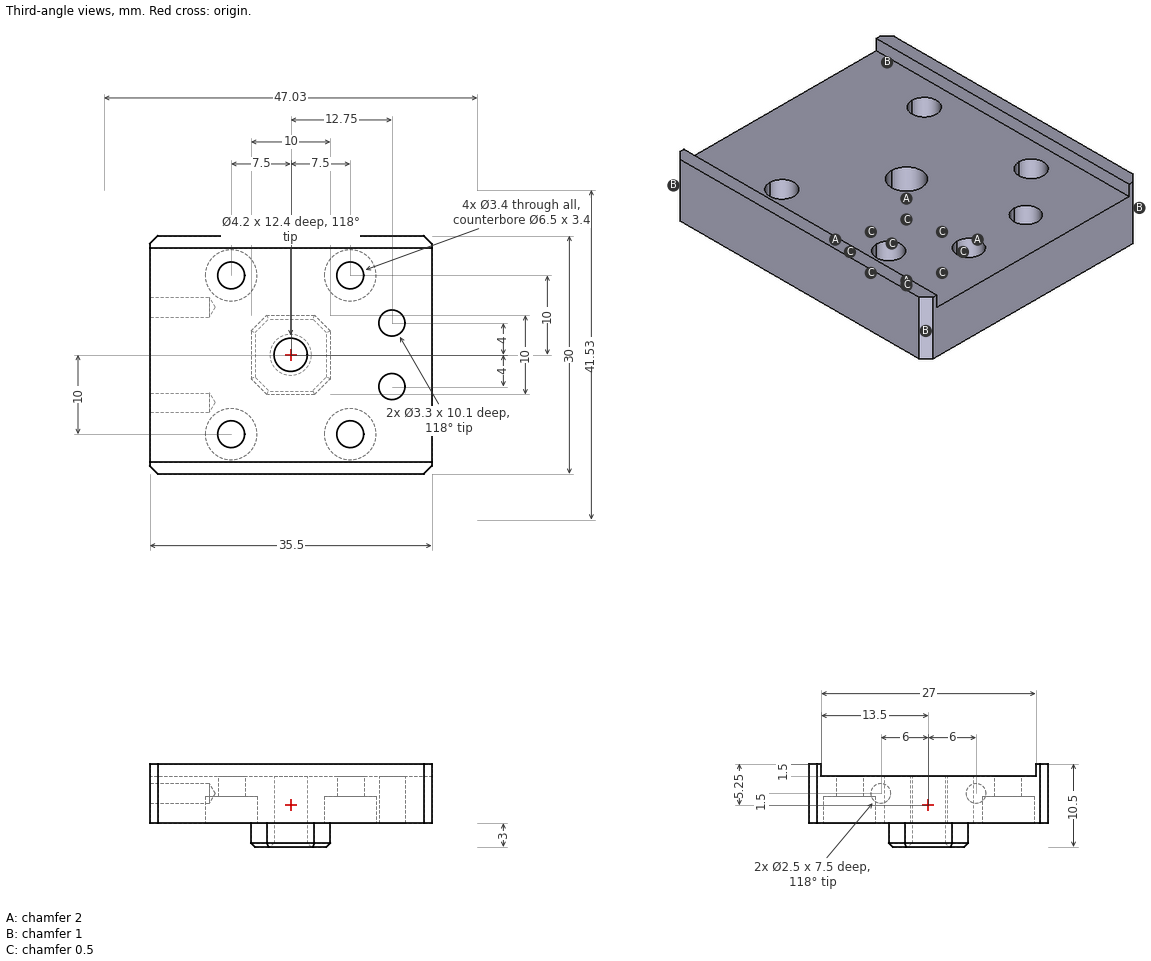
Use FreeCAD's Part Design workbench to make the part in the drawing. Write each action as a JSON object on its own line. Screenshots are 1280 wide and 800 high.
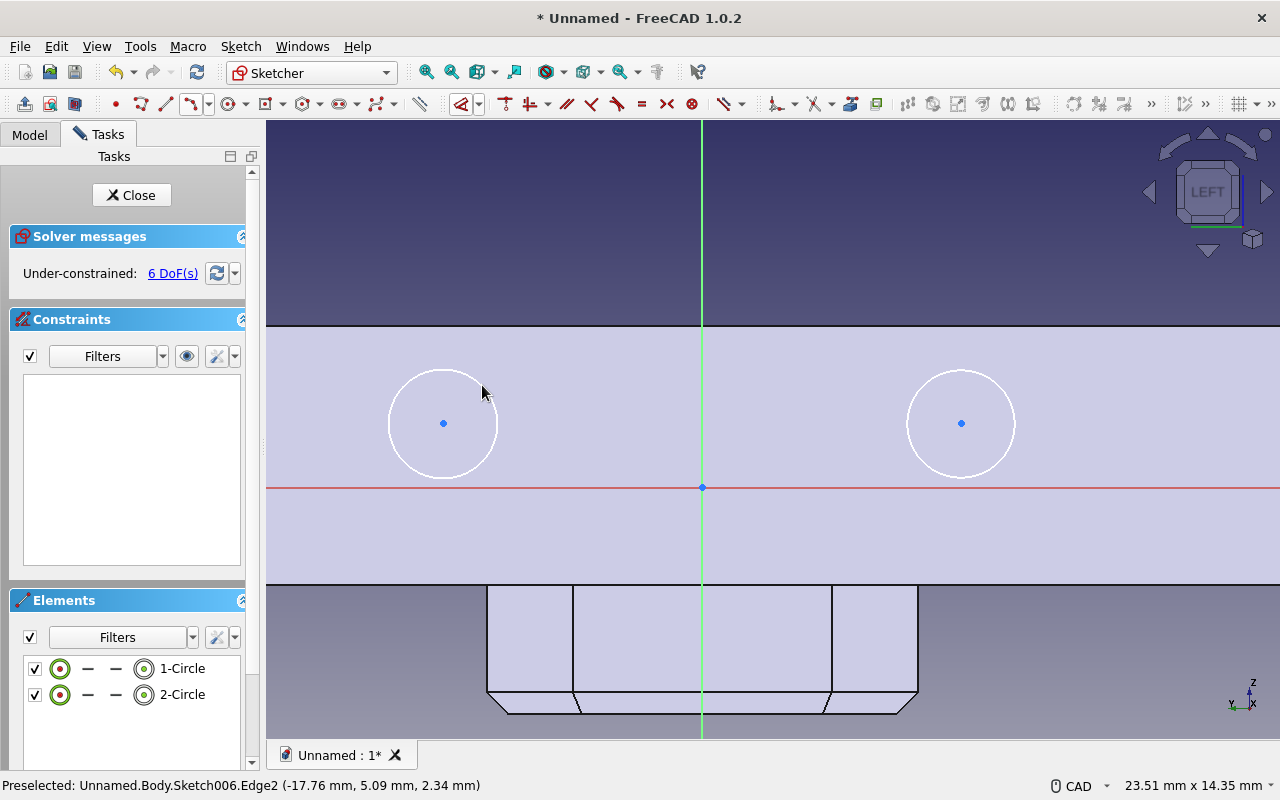
{"action": "left_click", "coordinate": [999, 386]}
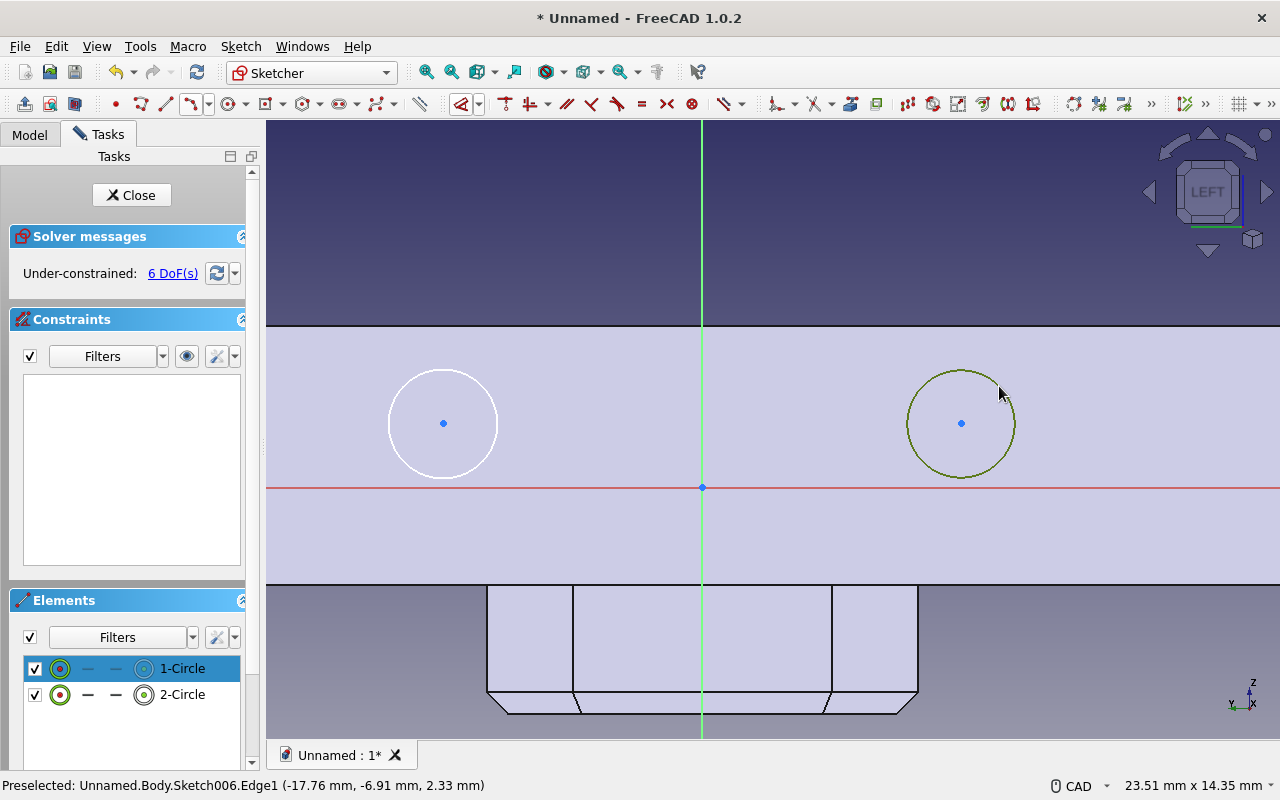
{"action": "left_click", "coordinate": [481, 385]}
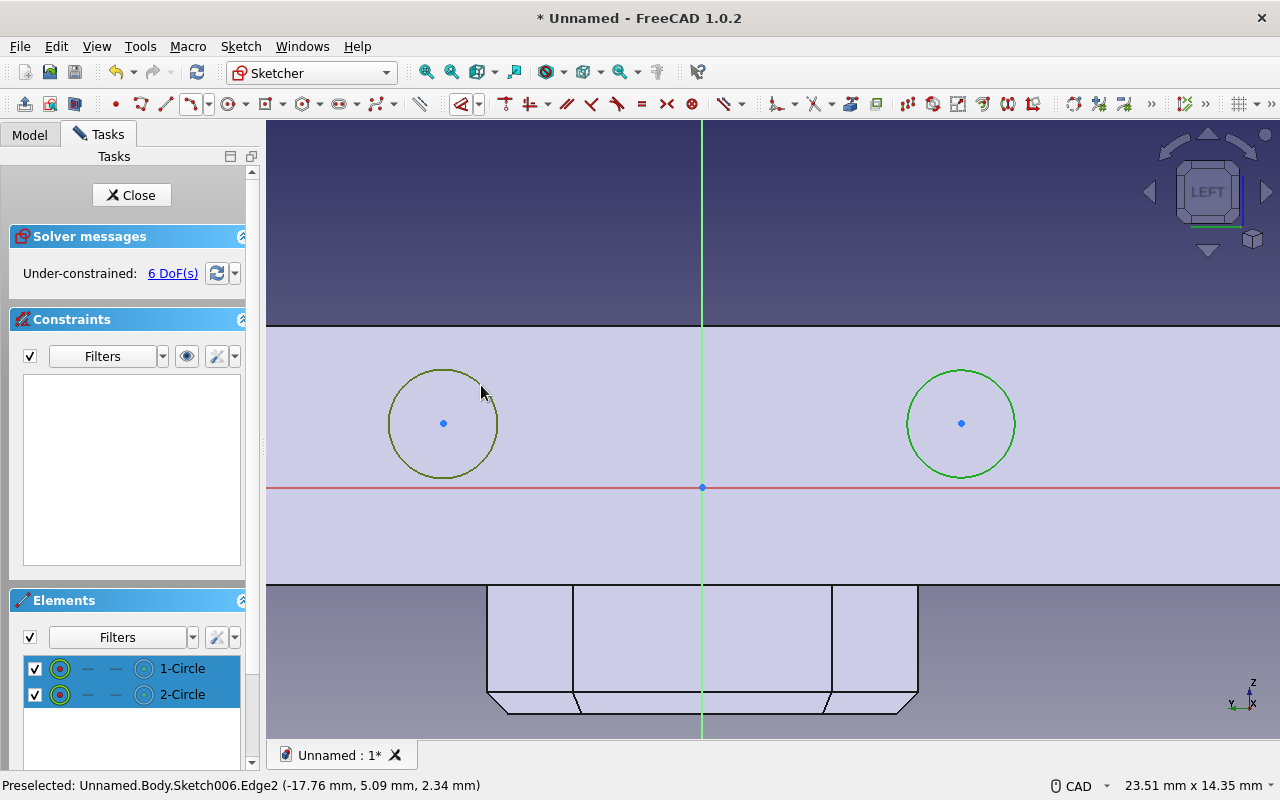
{"action": "key", "text": "e"}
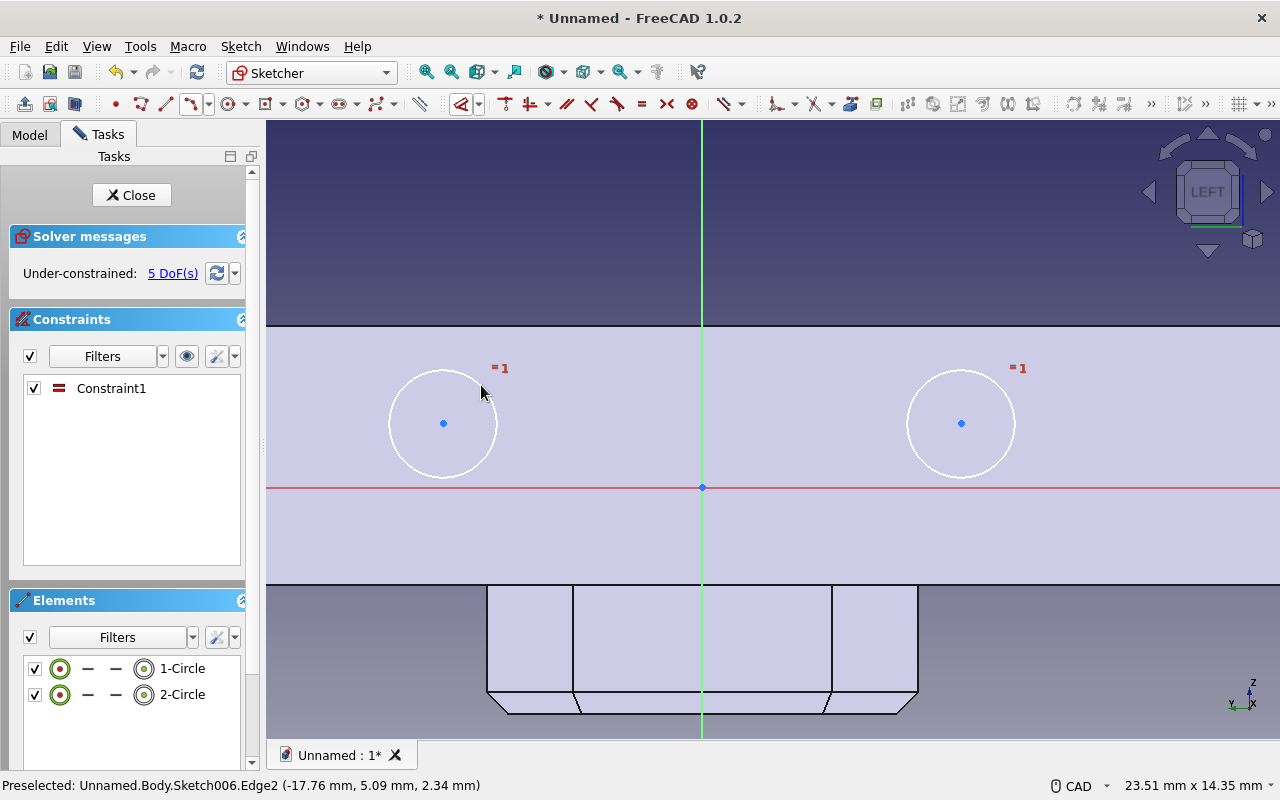
{"action": "left_click", "coordinate": [961, 424]}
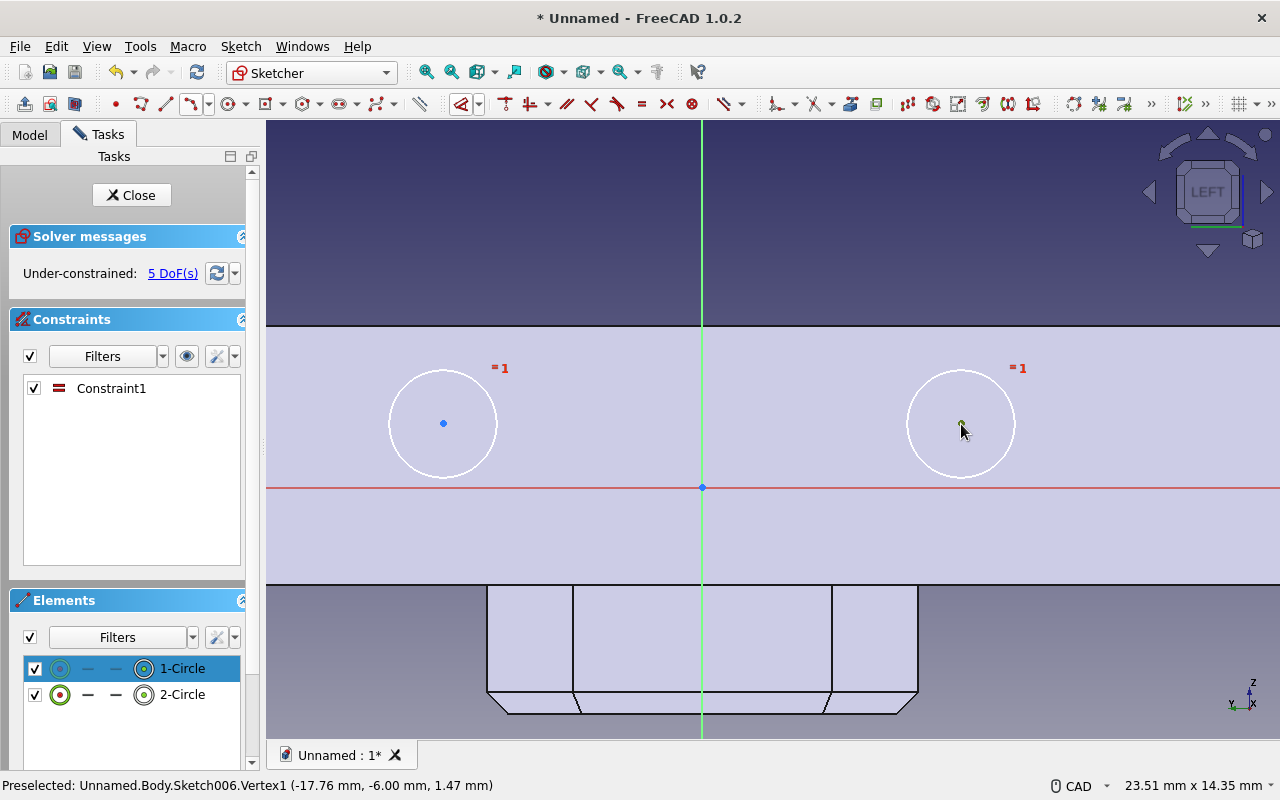
{"action": "left_click", "coordinate": [443, 424]}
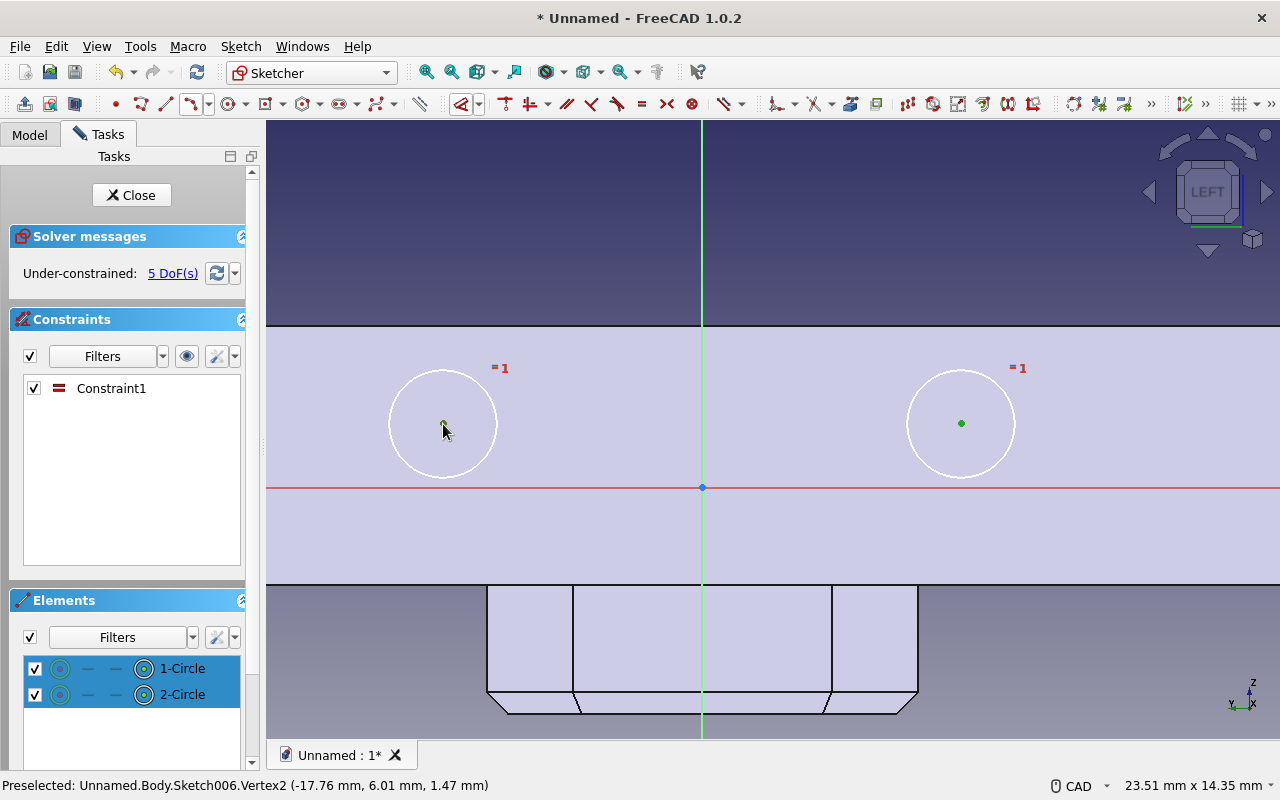
{"action": "key", "text": "h"}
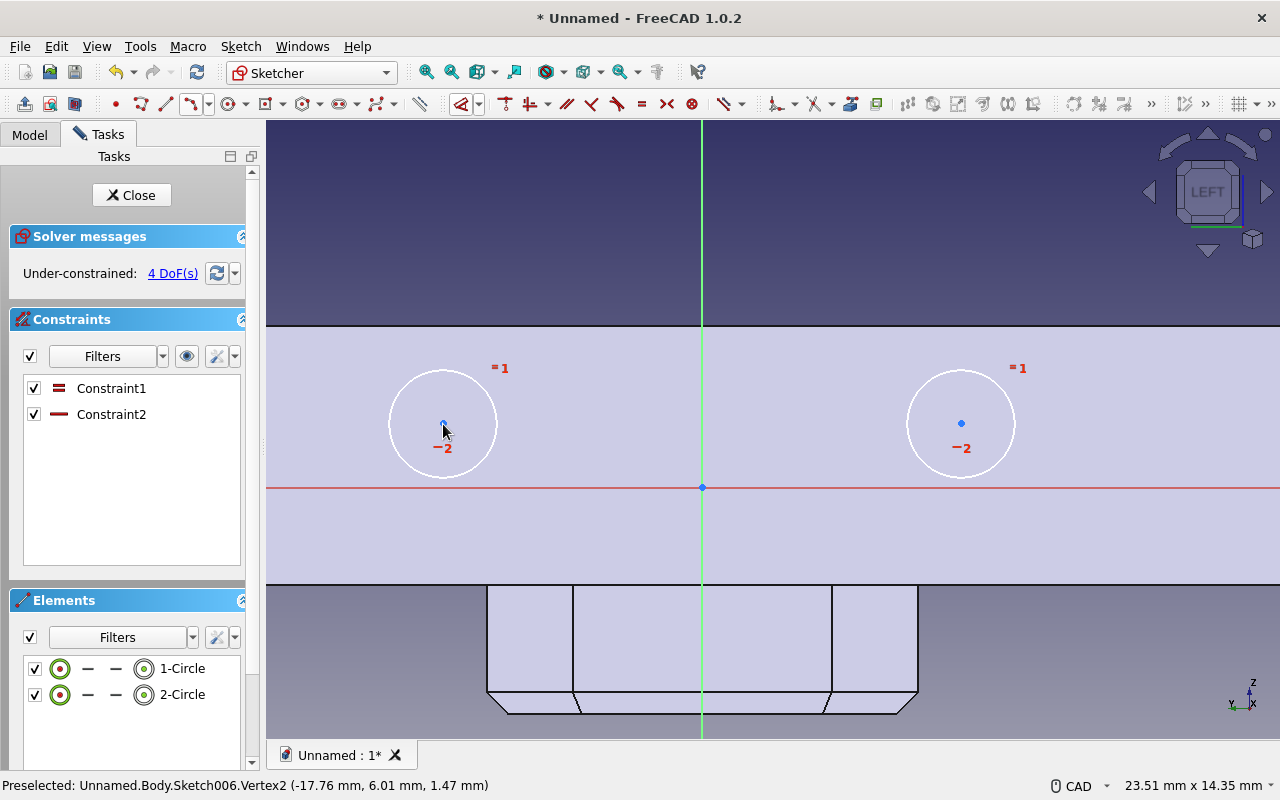
{"action": "left_click", "coordinate": [460, 104]}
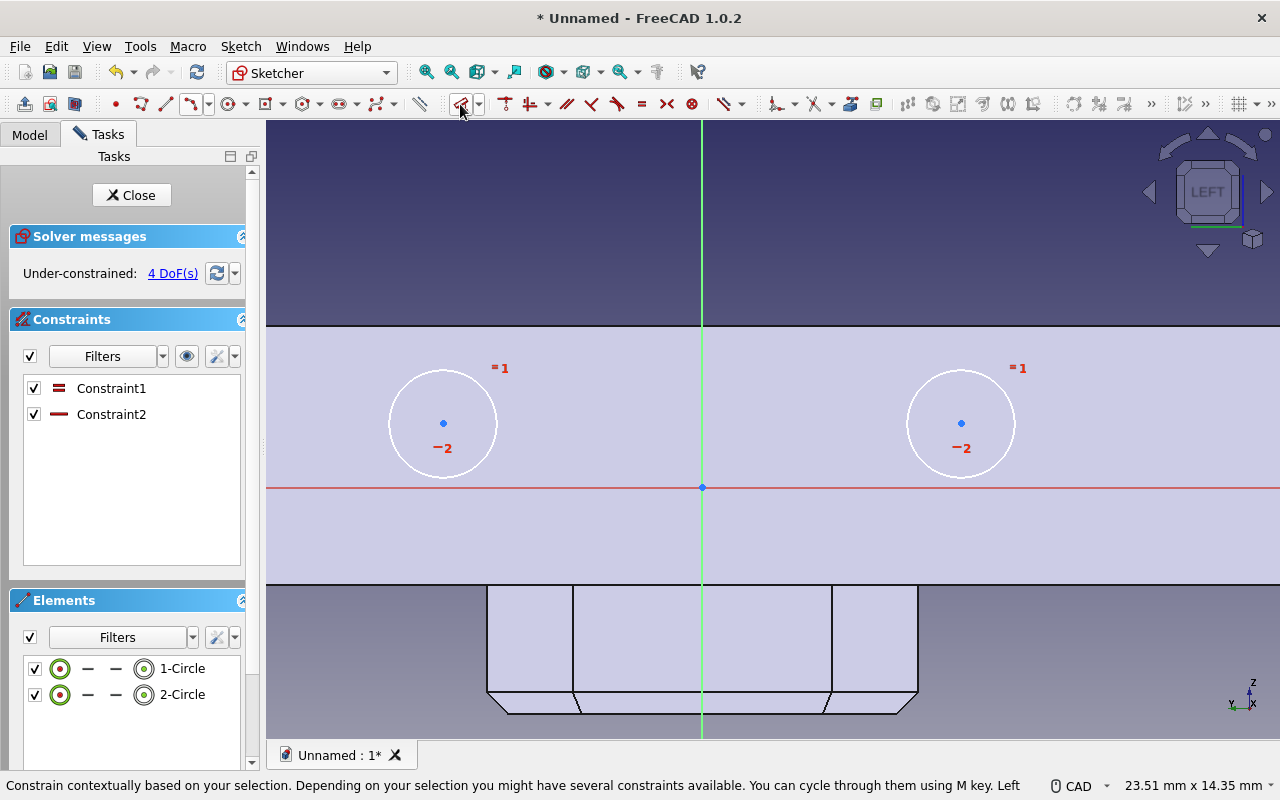
{"action": "left_click", "coordinate": [999, 386]}
{"action": "left_click", "coordinate": [1022, 363]}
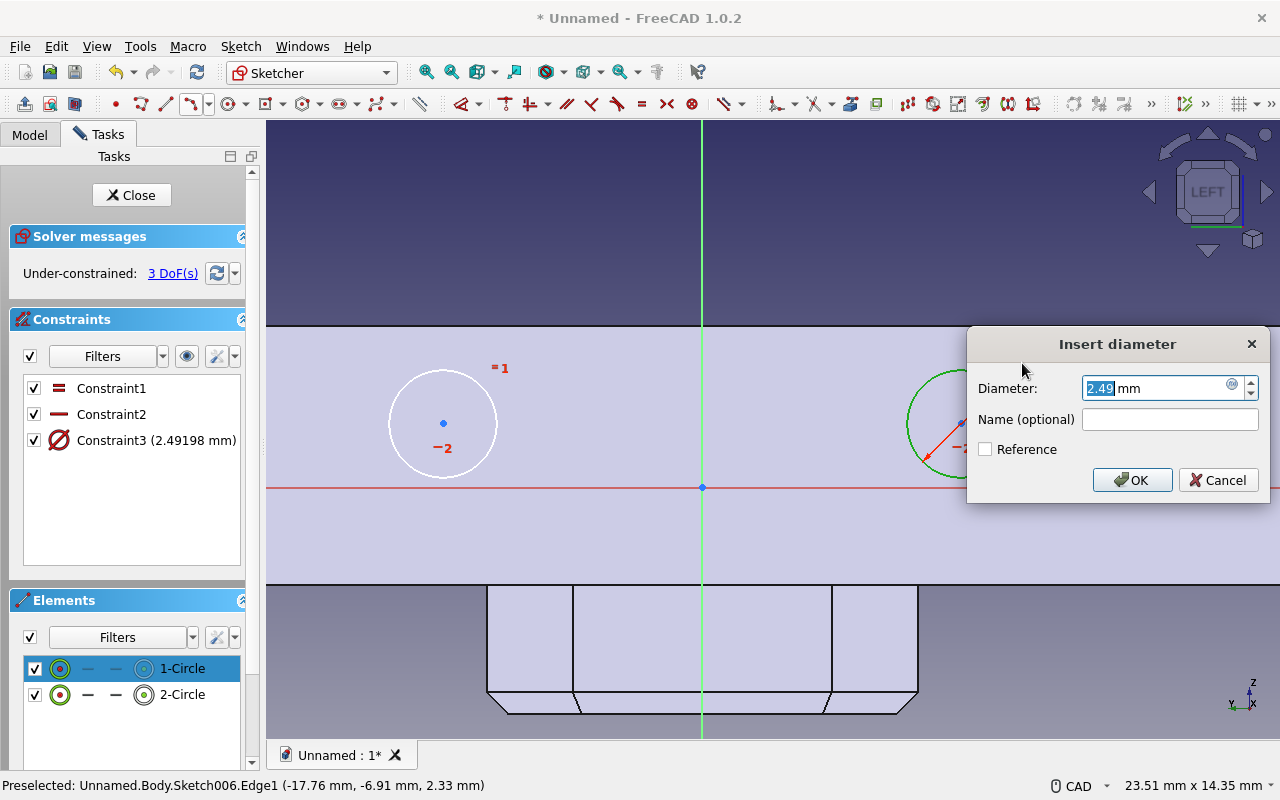
{"action": "type", "text": "2.5"}
{"action": "key", "text": "Return"}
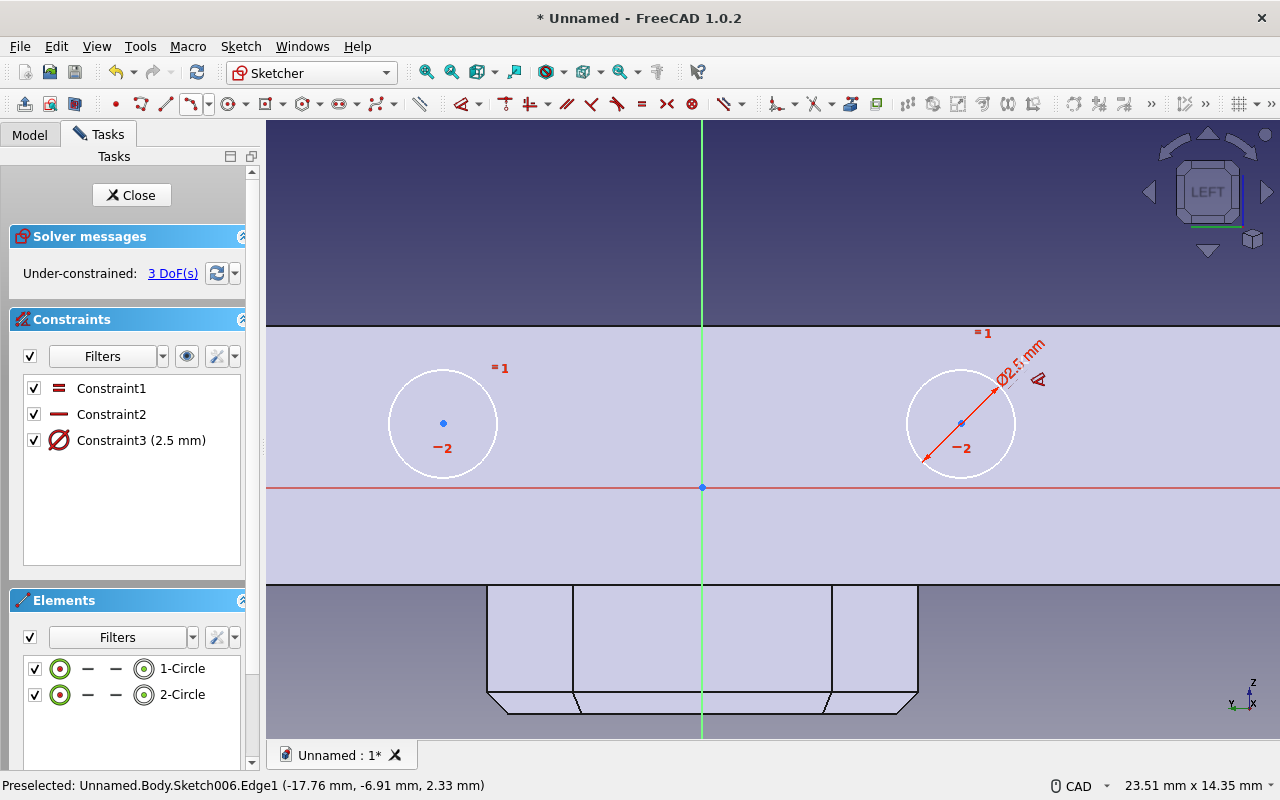
{"action": "left_click", "coordinate": [961, 424]}
{"action": "left_click", "coordinate": [832, 522]}